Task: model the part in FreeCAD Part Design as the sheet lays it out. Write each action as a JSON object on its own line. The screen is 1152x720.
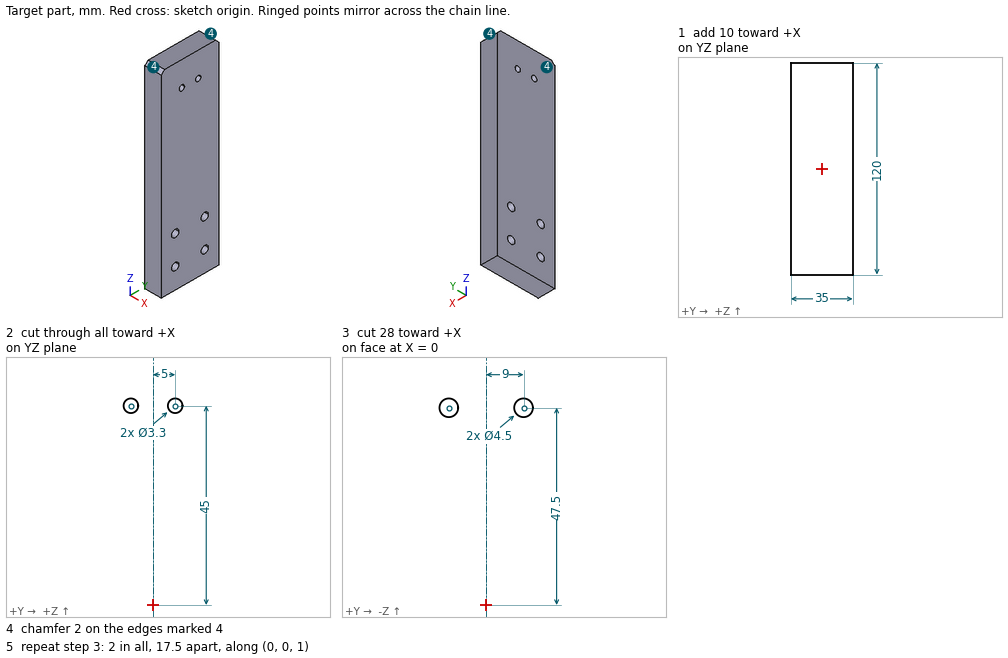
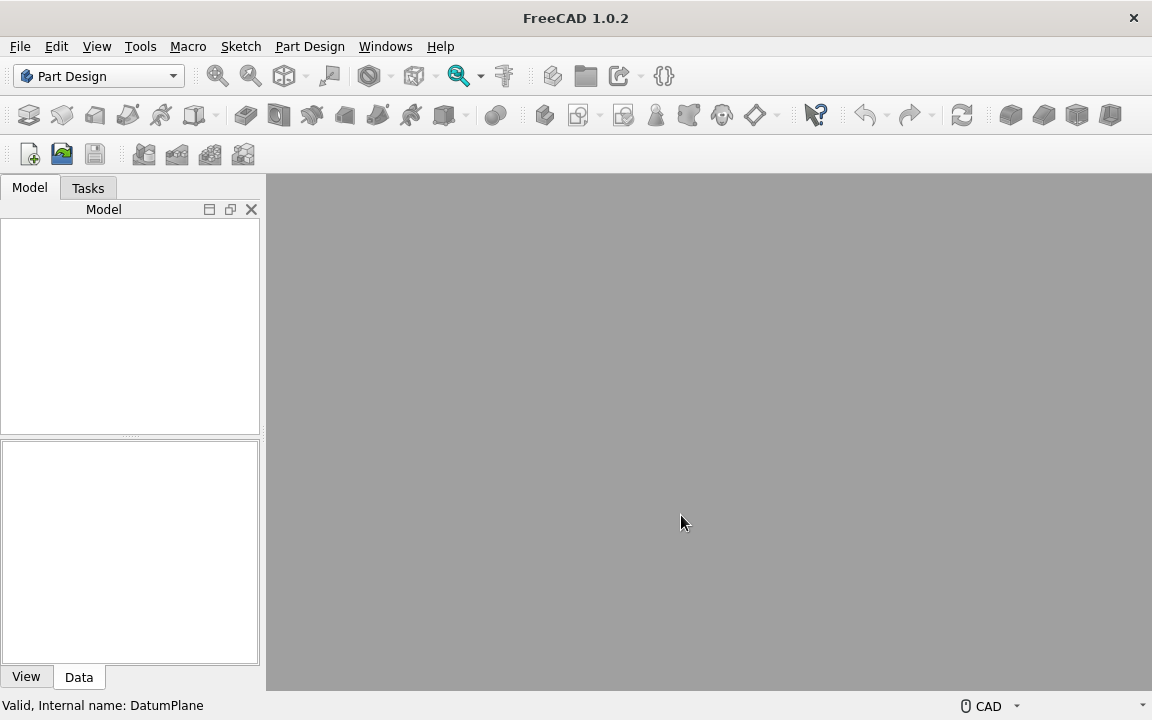
{"action": "left_click", "coordinate": [29, 154]}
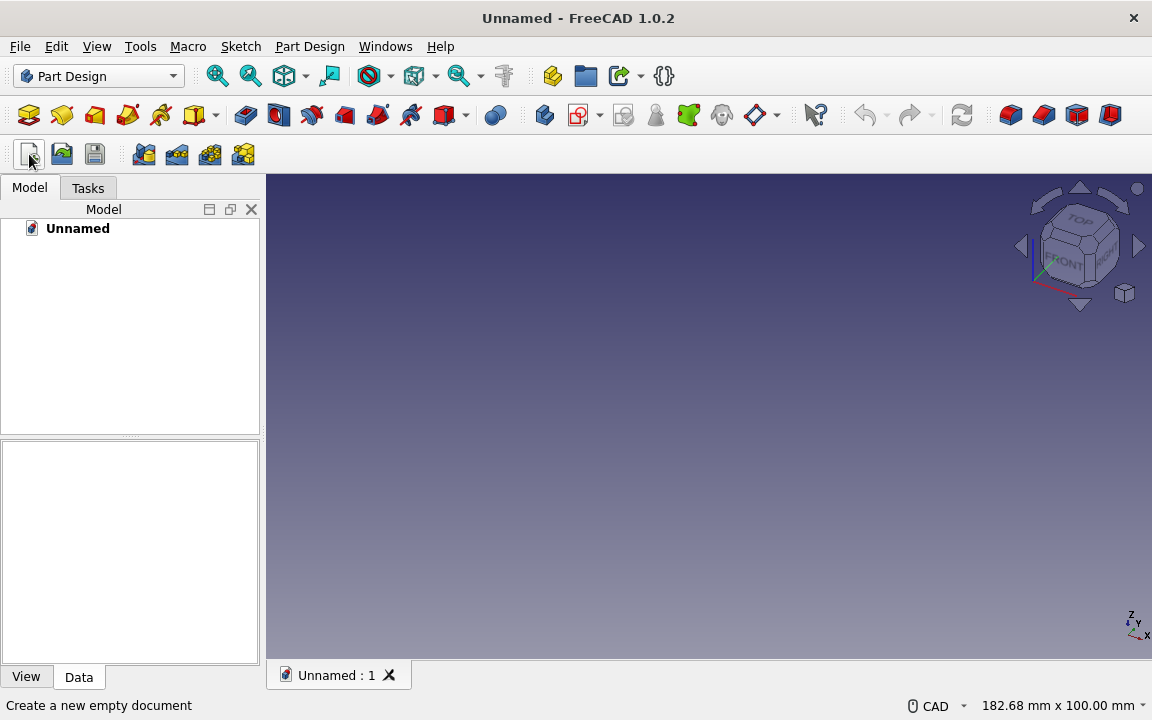
{"action": "left_click", "coordinate": [578, 116]}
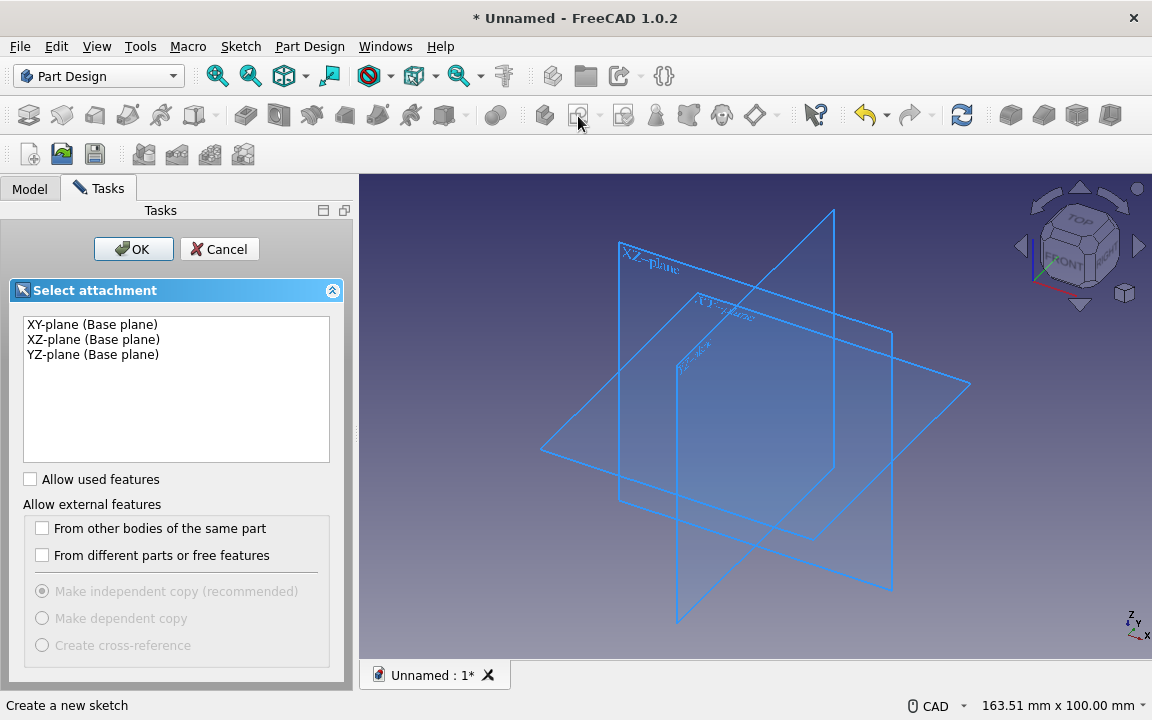
{"action": "left_click", "coordinate": [84, 354]}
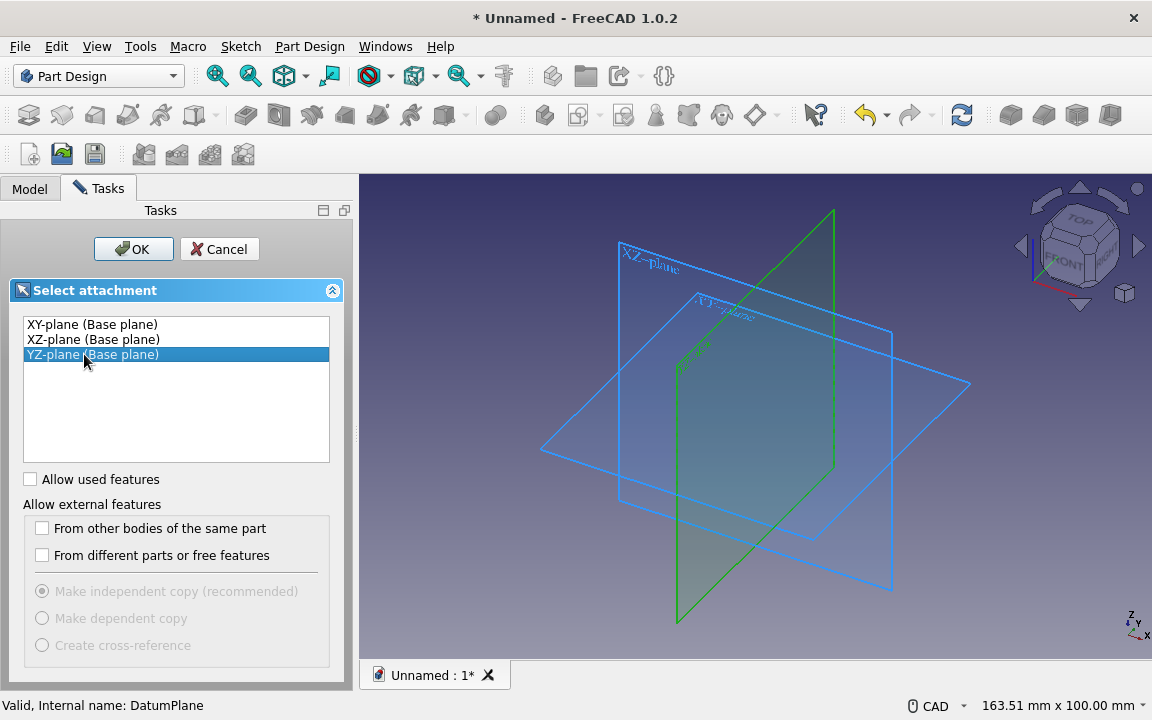
{"action": "left_click", "coordinate": [134, 249]}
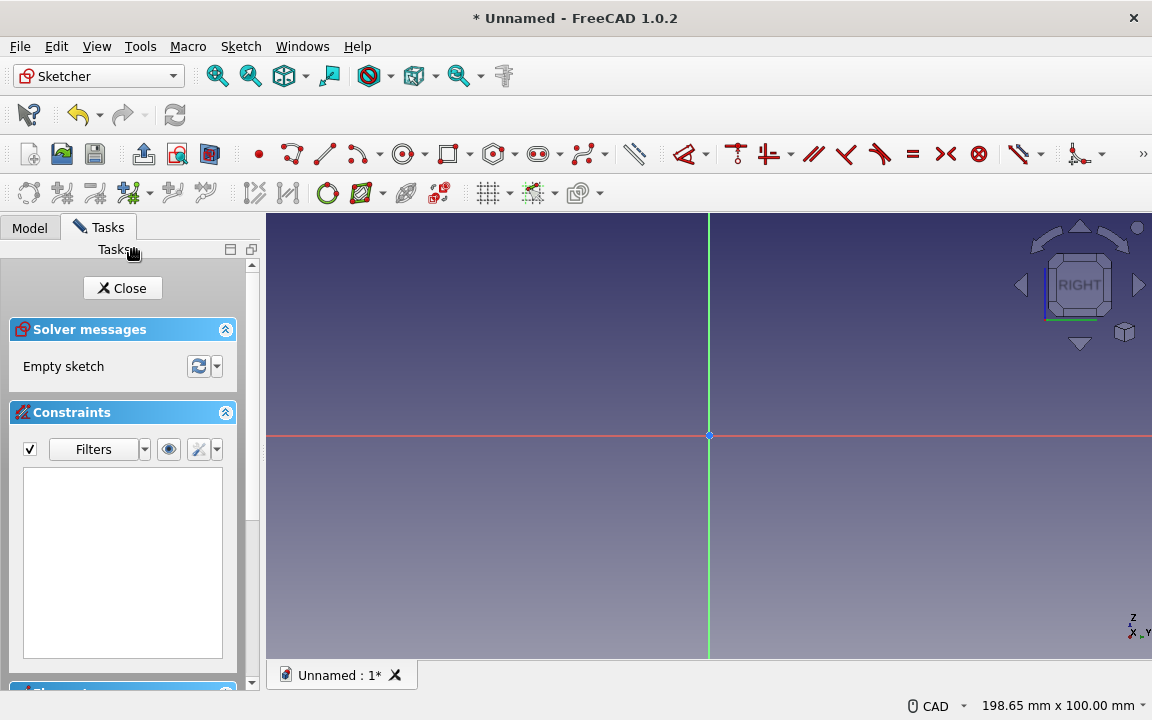
{"action": "scroll", "coordinate": [557, 436], "scroll_direction": "down", "scroll_amount": 3}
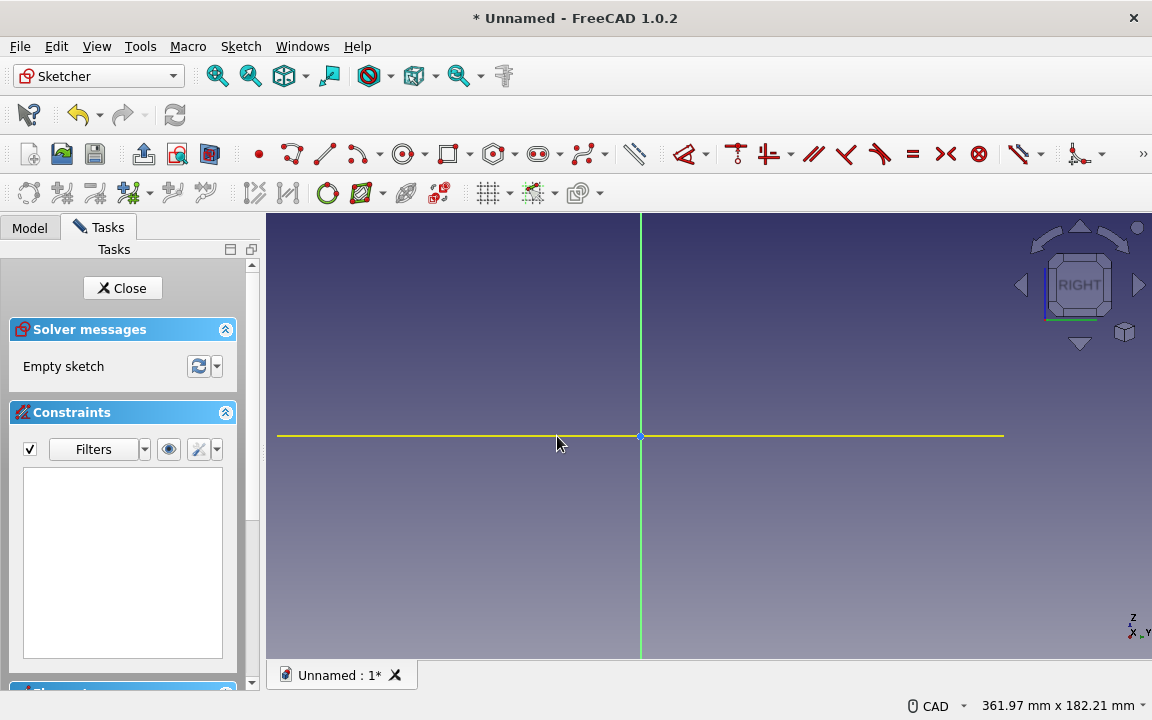
{"action": "key", "text": "g v"}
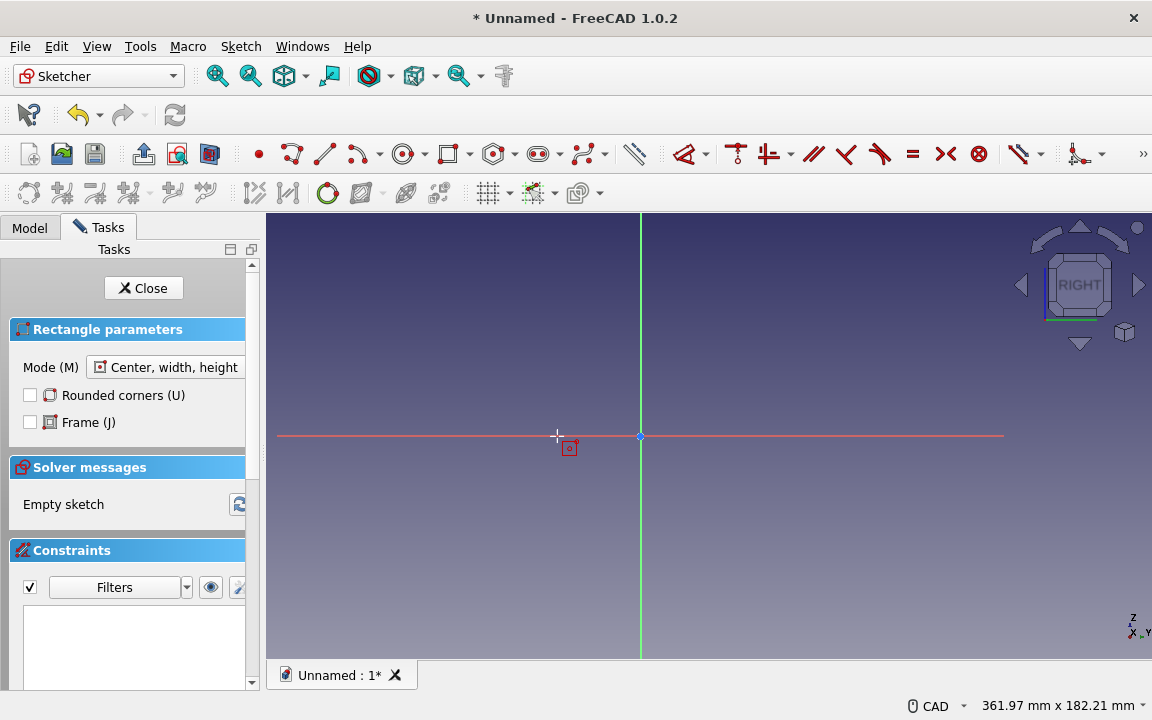
{"action": "left_click", "coordinate": [641, 436]}
{"action": "left_click", "coordinate": [683, 289]}
{"action": "key", "text": "Escape"}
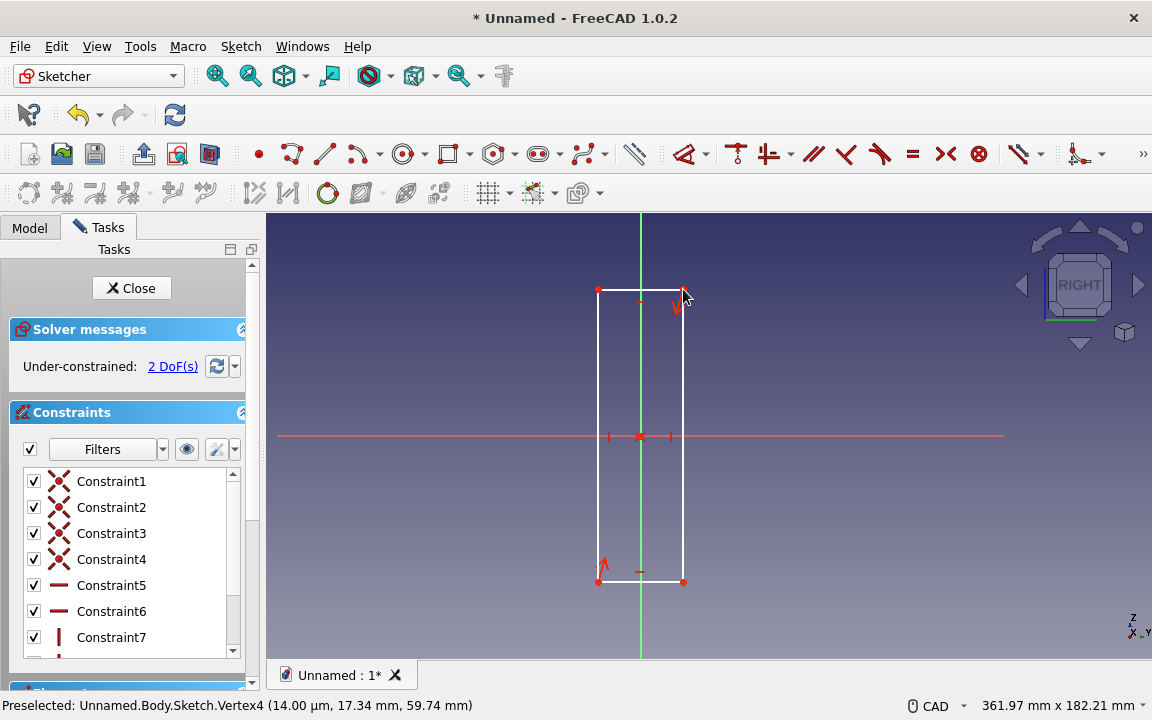
{"action": "left_click", "coordinate": [684, 154]}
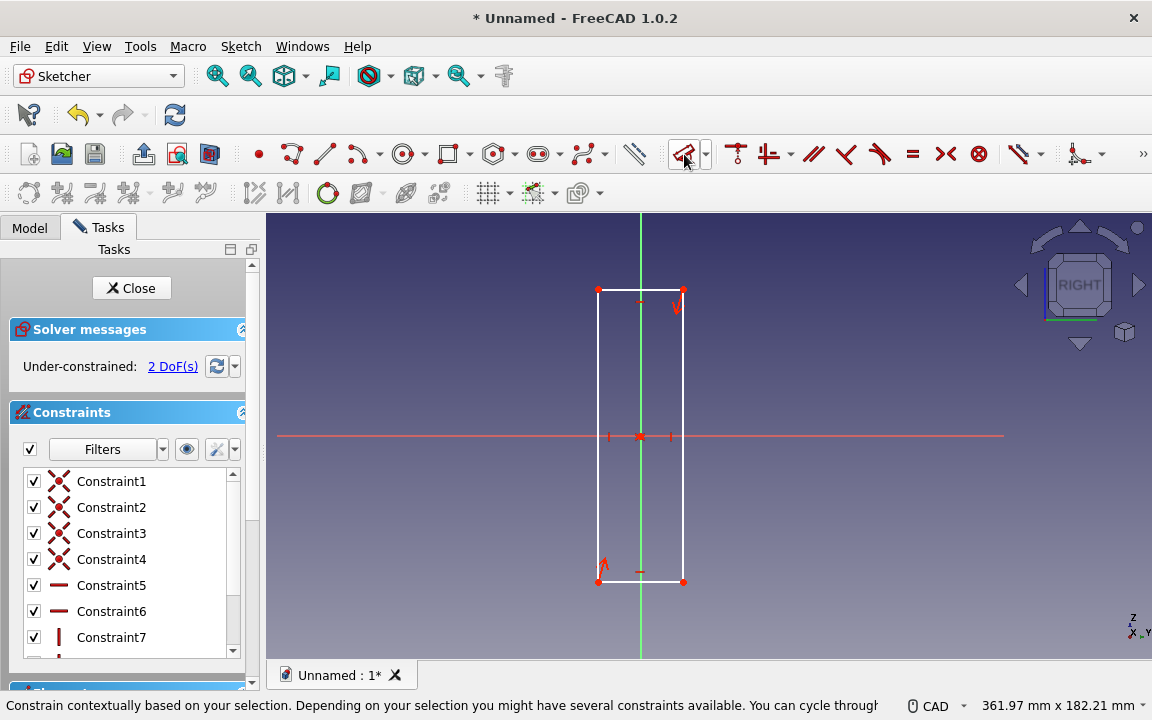
{"action": "left_click", "coordinate": [624, 582]}
{"action": "left_click", "coordinate": [621, 616]}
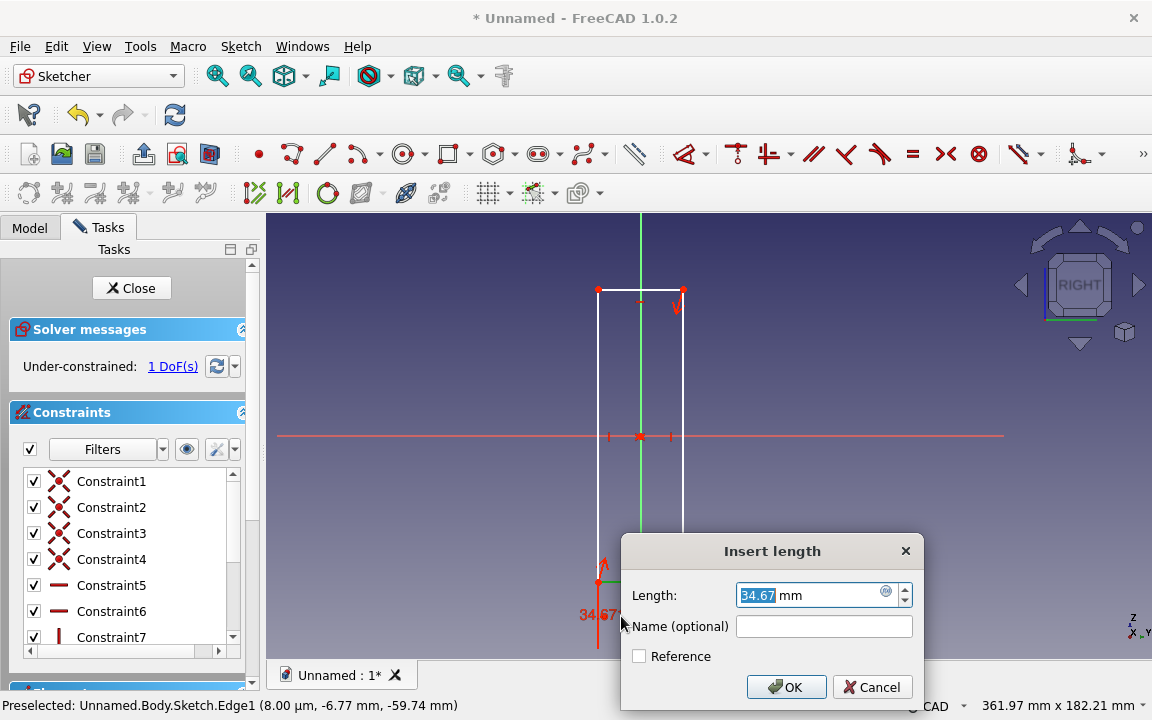
{"action": "type", "text": "35"}
{"action": "key", "text": "Return"}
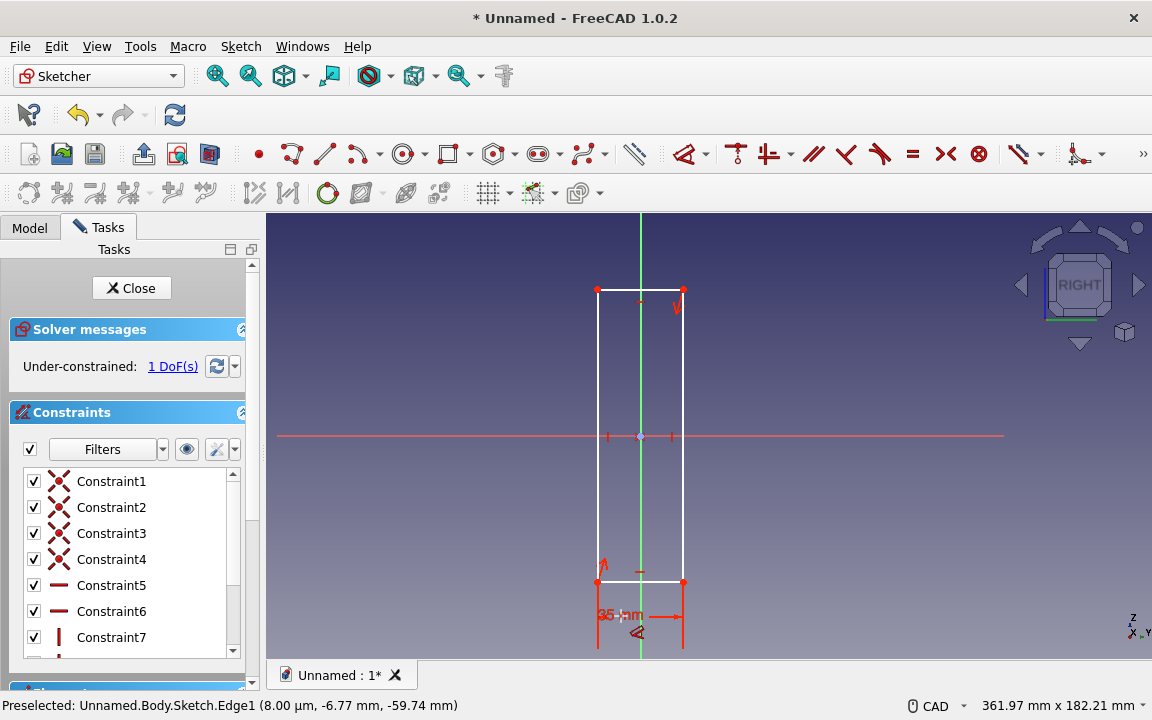
{"action": "left_click", "coordinate": [683, 495]}
{"action": "left_click", "coordinate": [717, 369]}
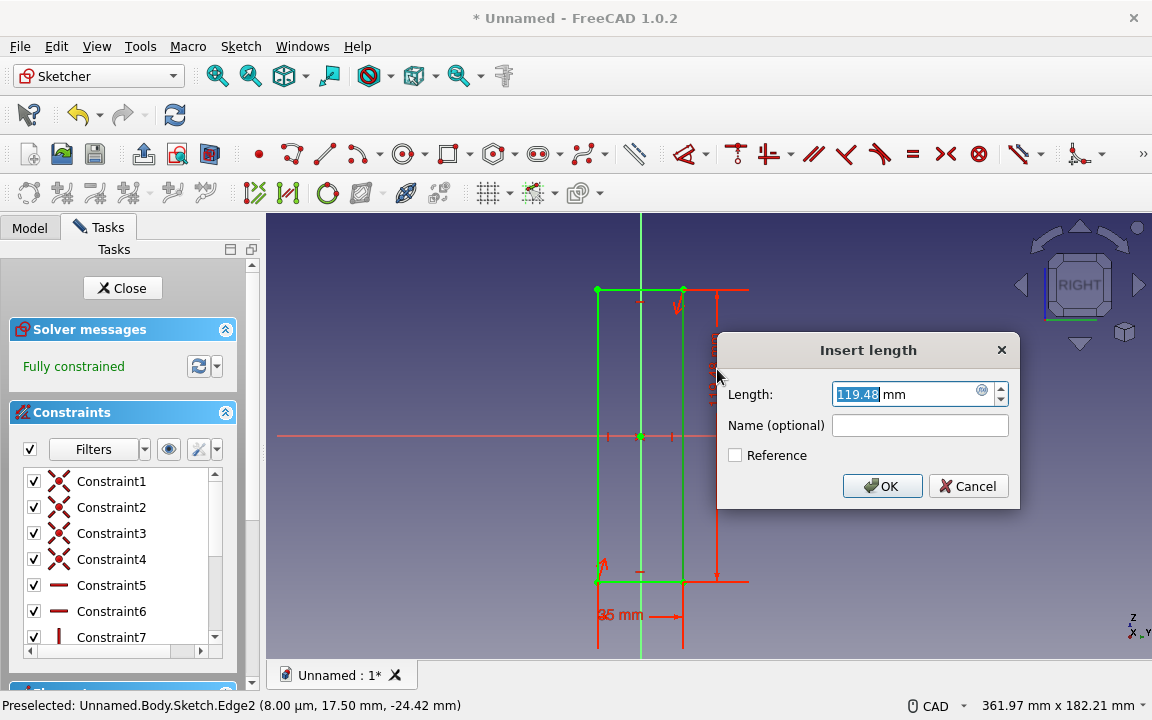
{"action": "type", "text": "120"}
{"action": "key", "text": "Return"}
{"action": "key", "text": "Escape"}